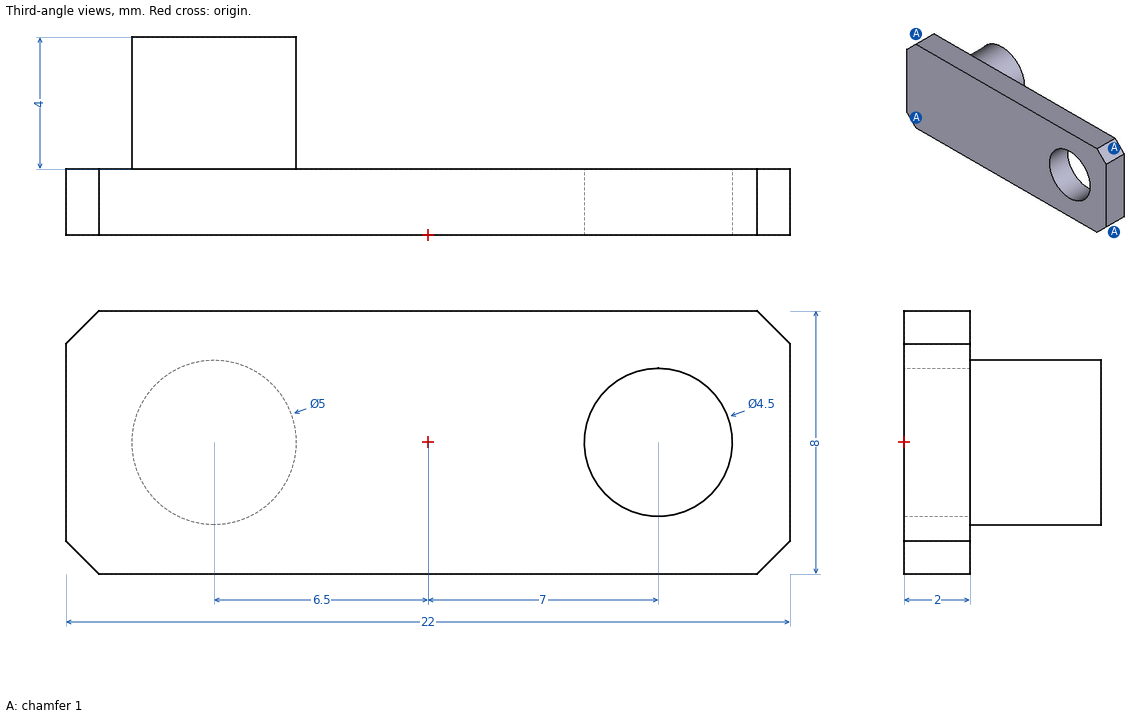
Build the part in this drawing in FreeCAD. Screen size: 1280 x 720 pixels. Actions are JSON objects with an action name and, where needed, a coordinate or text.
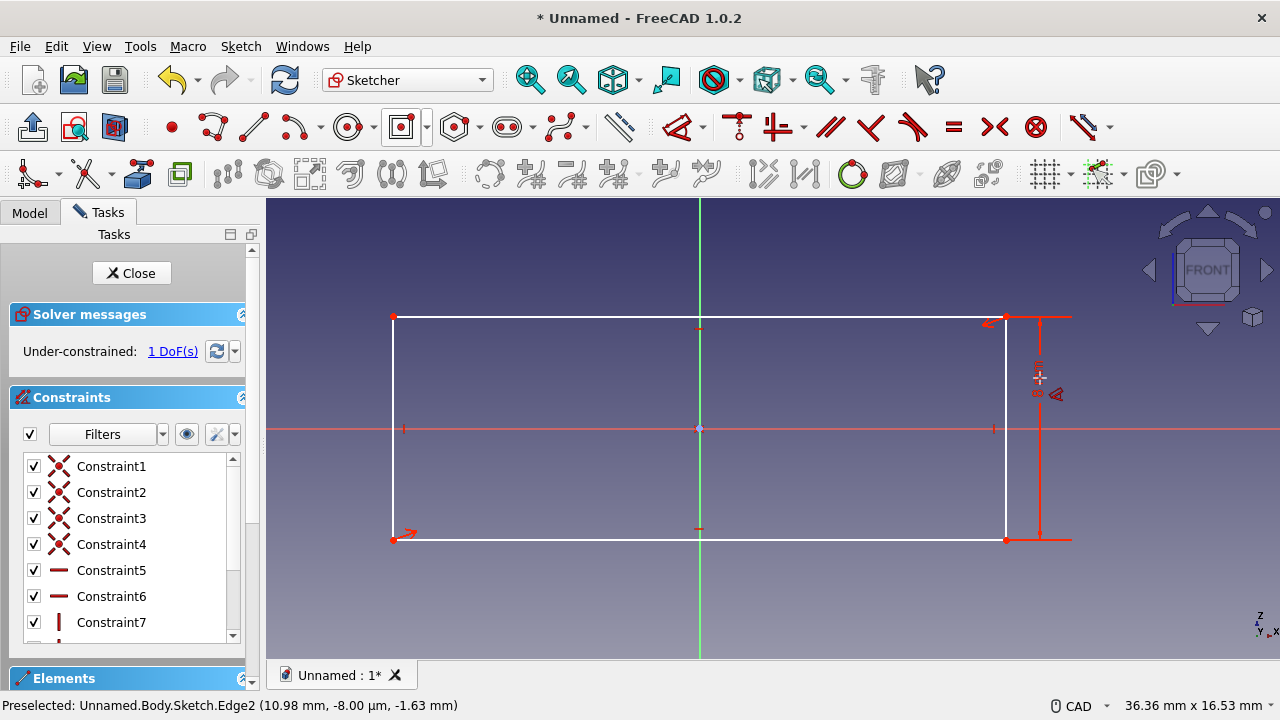
{"action": "left_click", "coordinate": [577, 540]}
{"action": "left_click", "coordinate": [559, 574]}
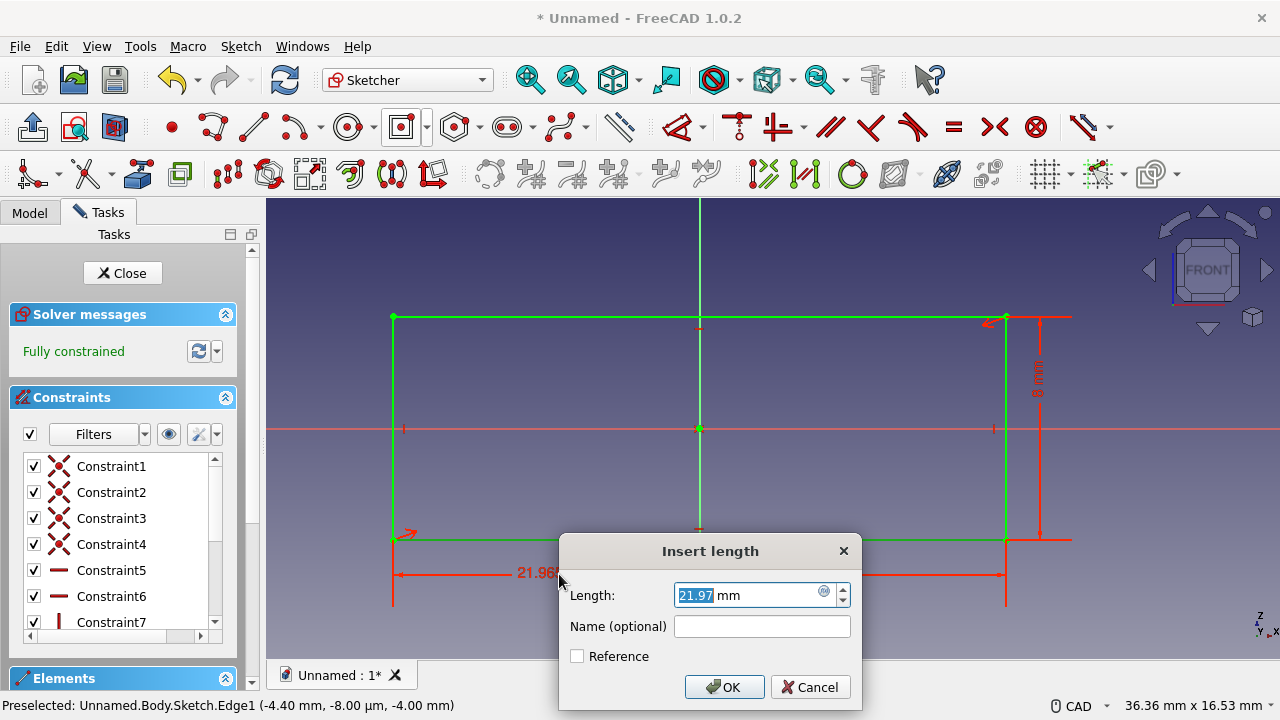
{"action": "type", "text": "22"}
{"action": "key", "text": "Return"}
{"action": "key", "text": "Escape"}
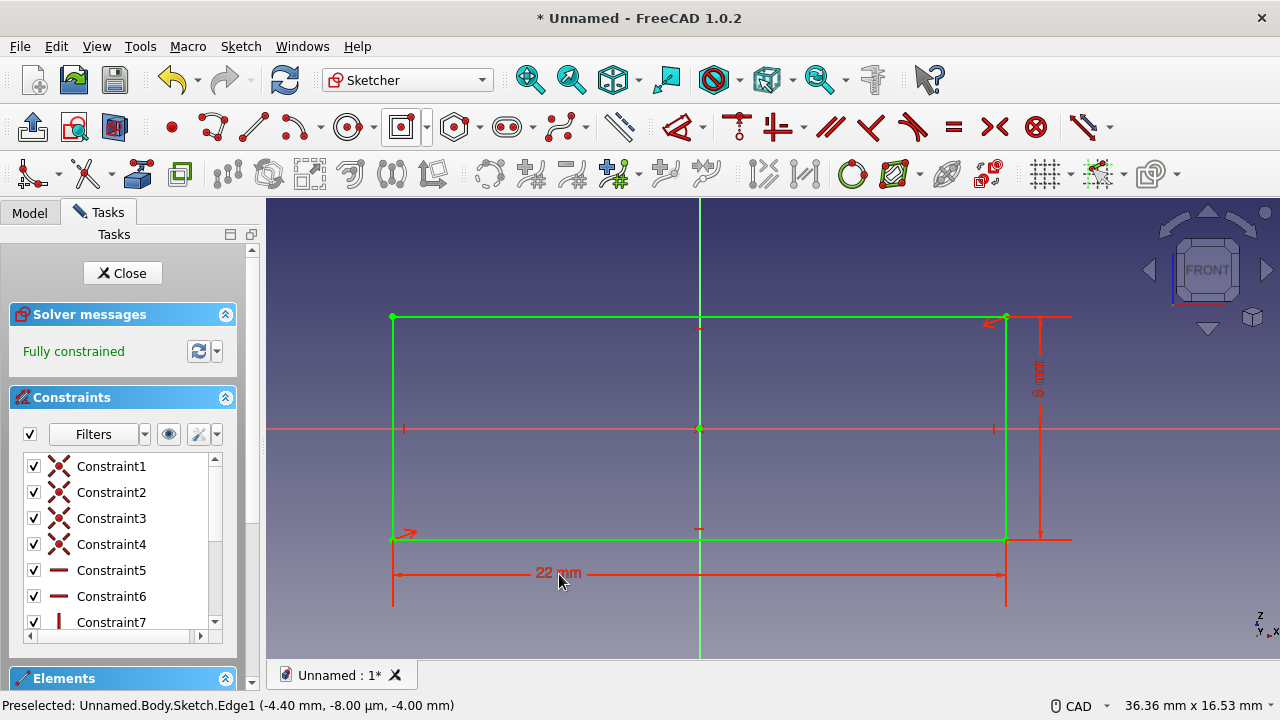
{"action": "left_click", "coordinate": [123, 273]}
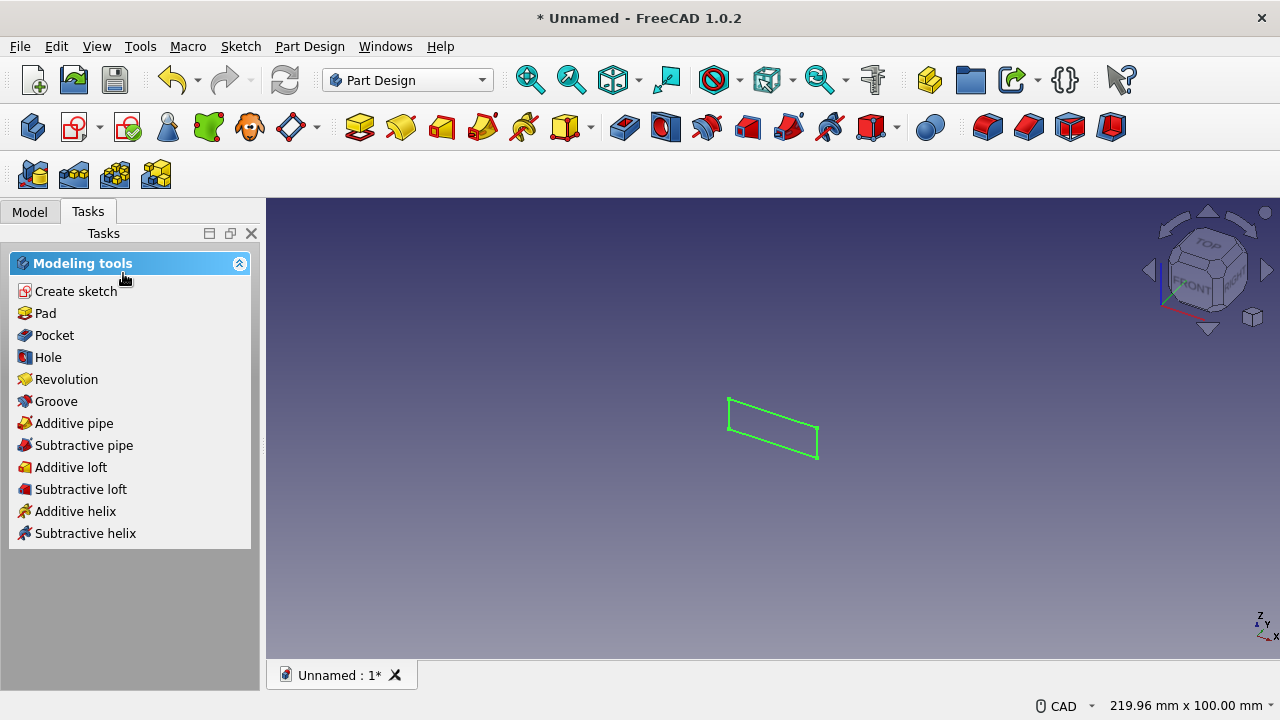
{"action": "left_click", "coordinate": [360, 128]}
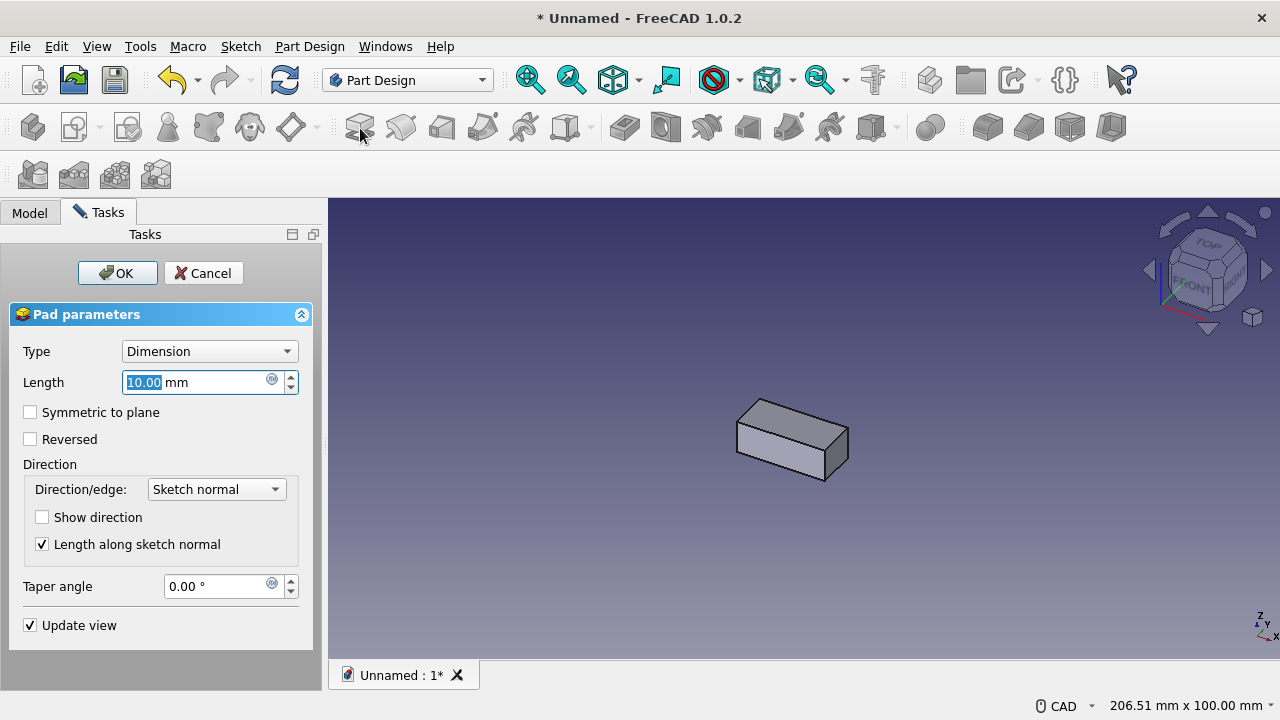
{"action": "type", "text": "2"}
{"action": "key", "text": "Tab"}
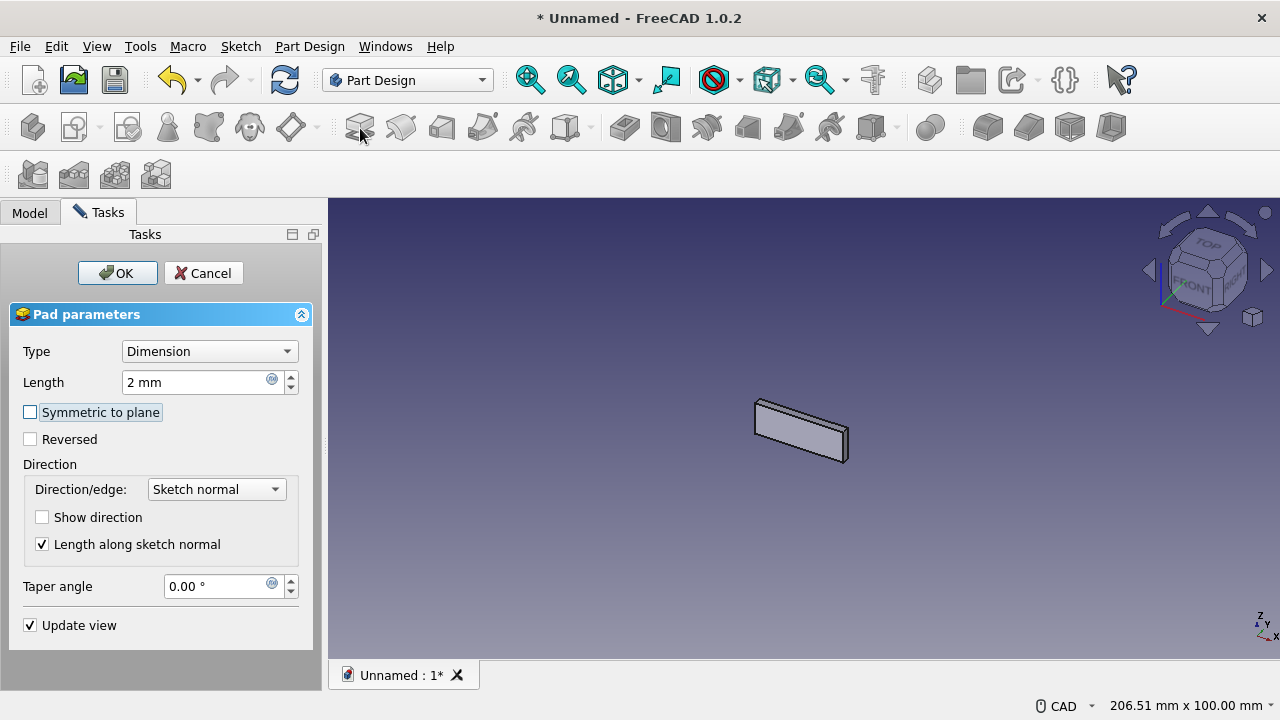
{"action": "left_click", "coordinate": [31, 439]}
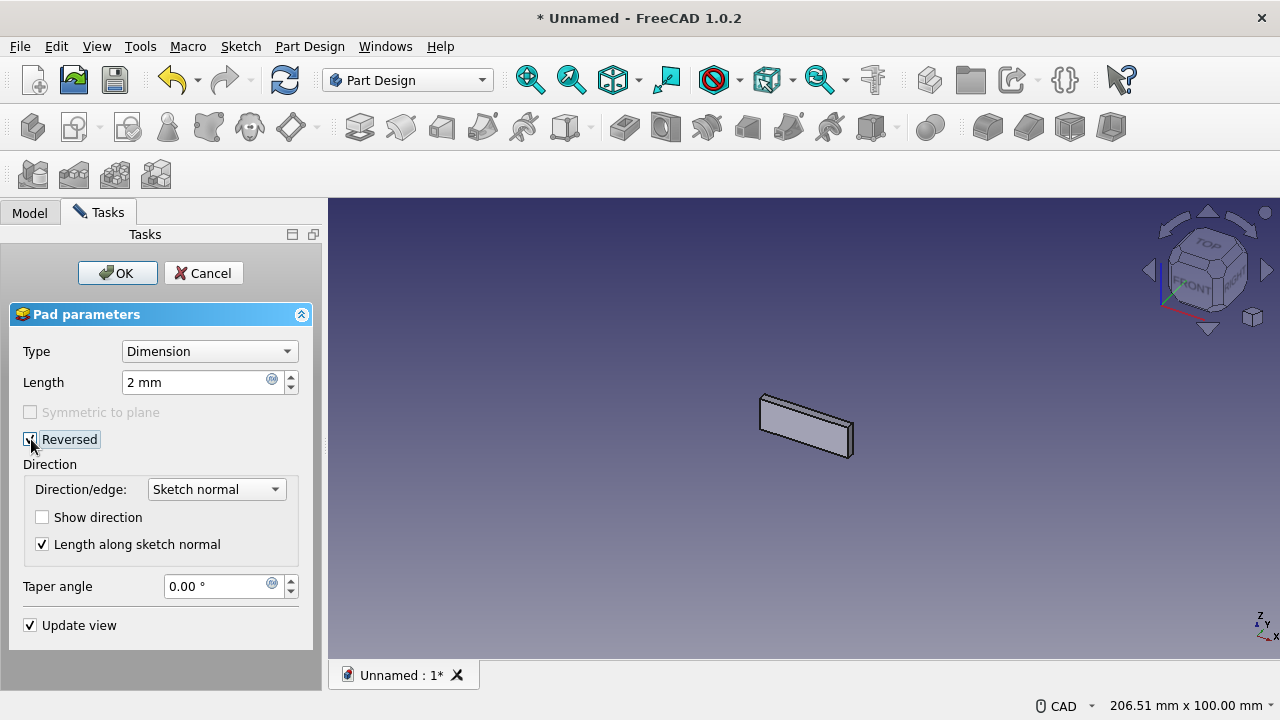
{"action": "left_click", "coordinate": [118, 273]}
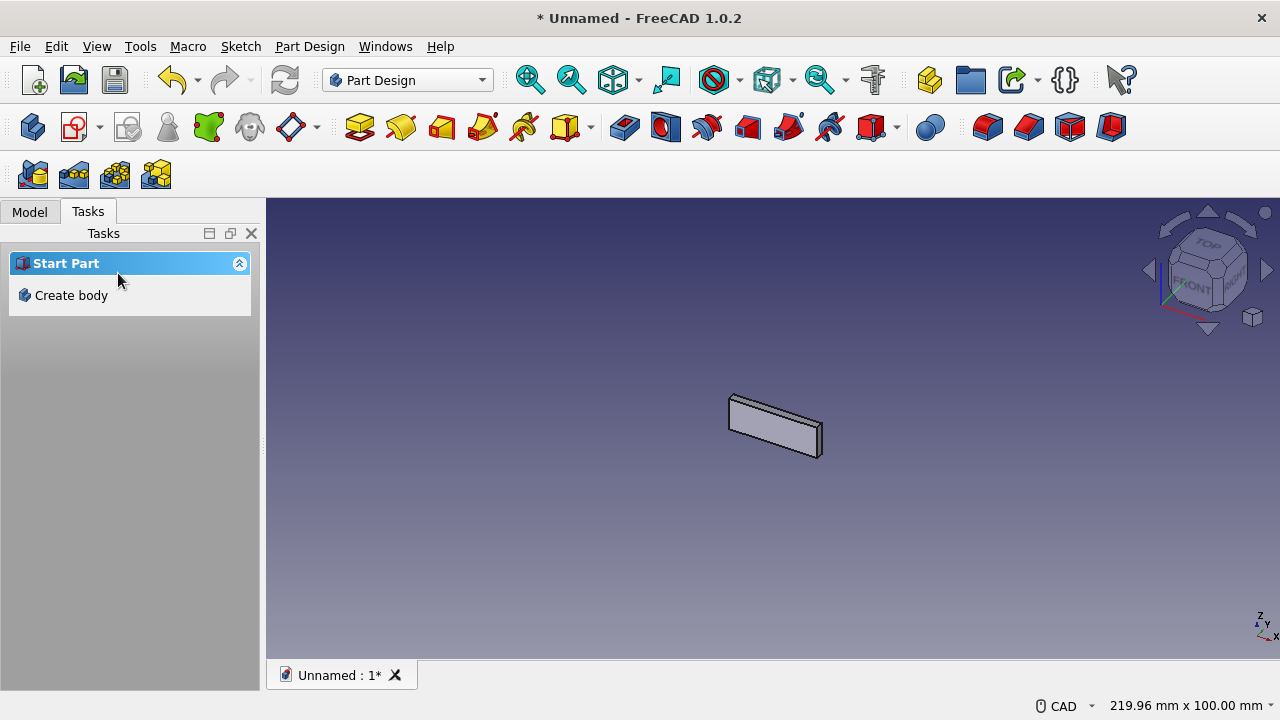
{"action": "left_click", "coordinate": [531, 80]}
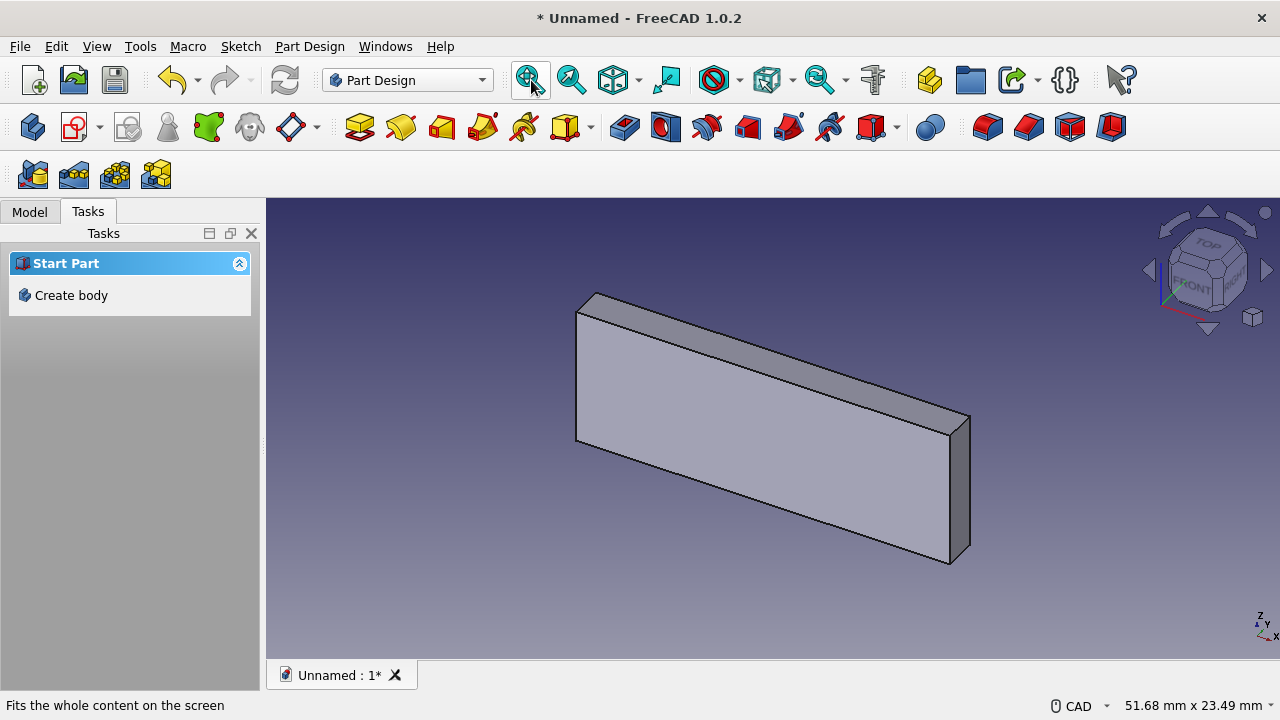
{"action": "key", "text": "4"}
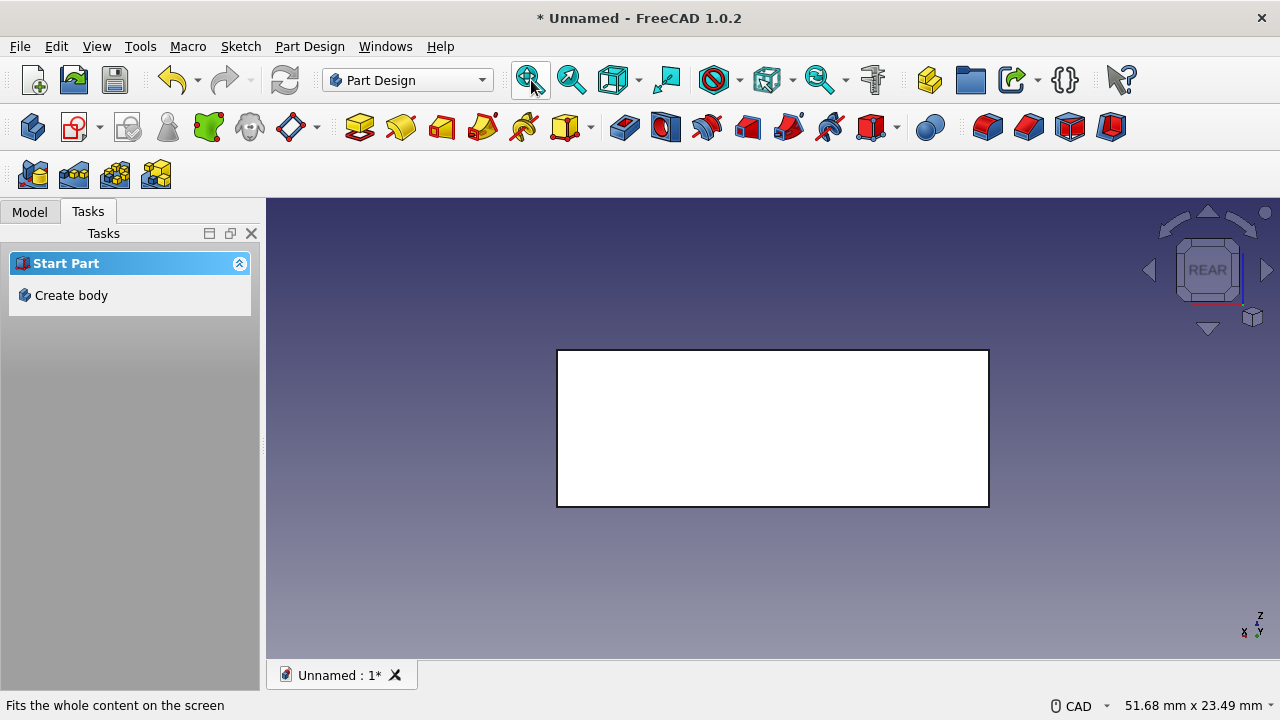
{"action": "left_click", "coordinate": [531, 80]}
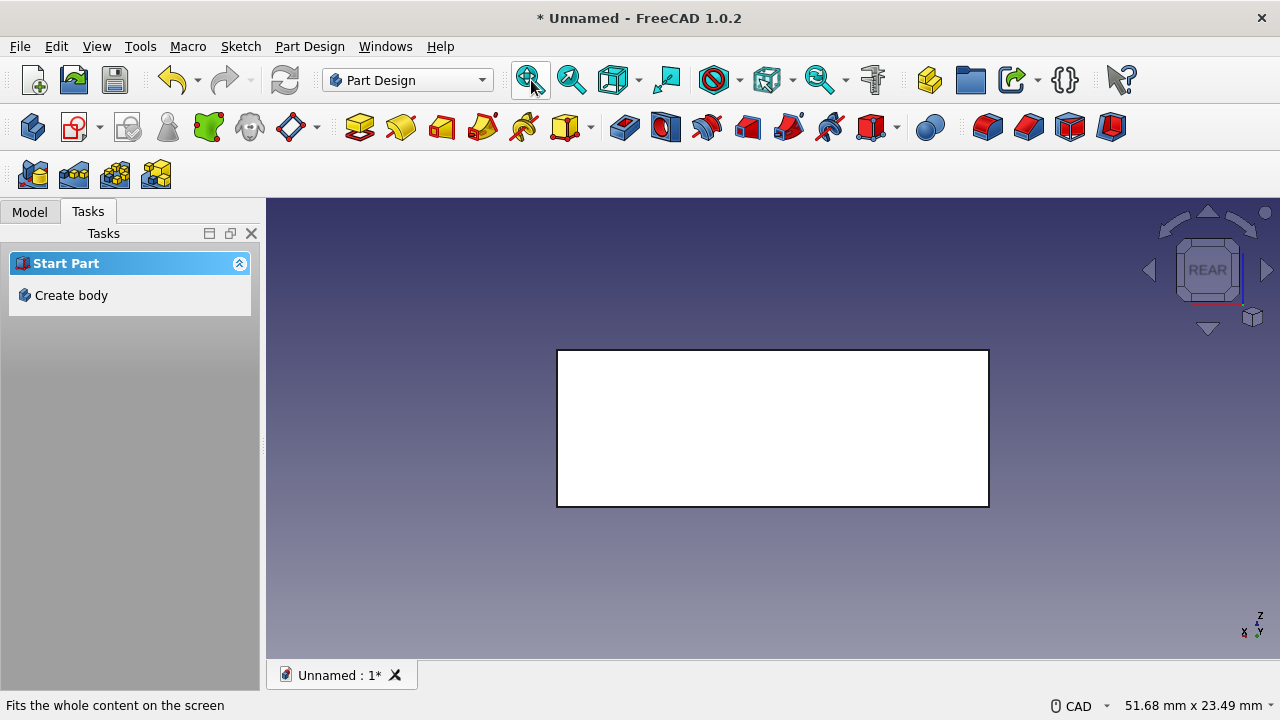
{"action": "left_click", "coordinate": [650, 428]}